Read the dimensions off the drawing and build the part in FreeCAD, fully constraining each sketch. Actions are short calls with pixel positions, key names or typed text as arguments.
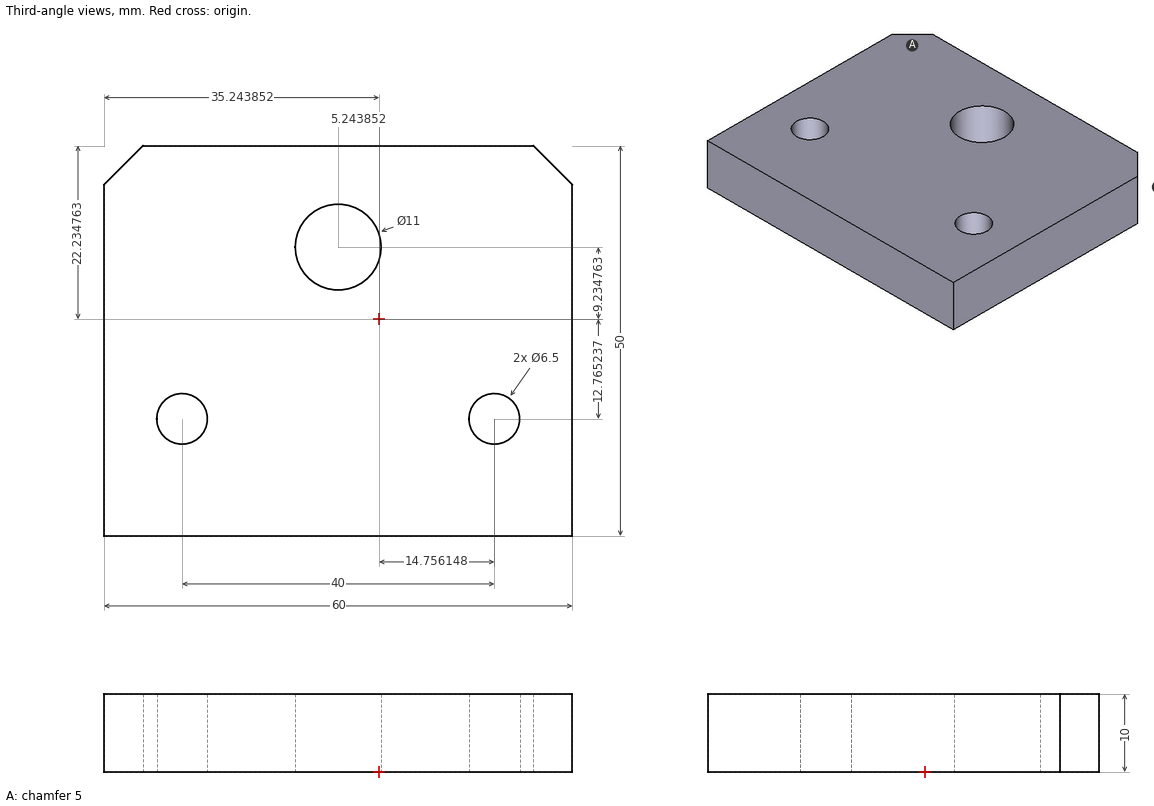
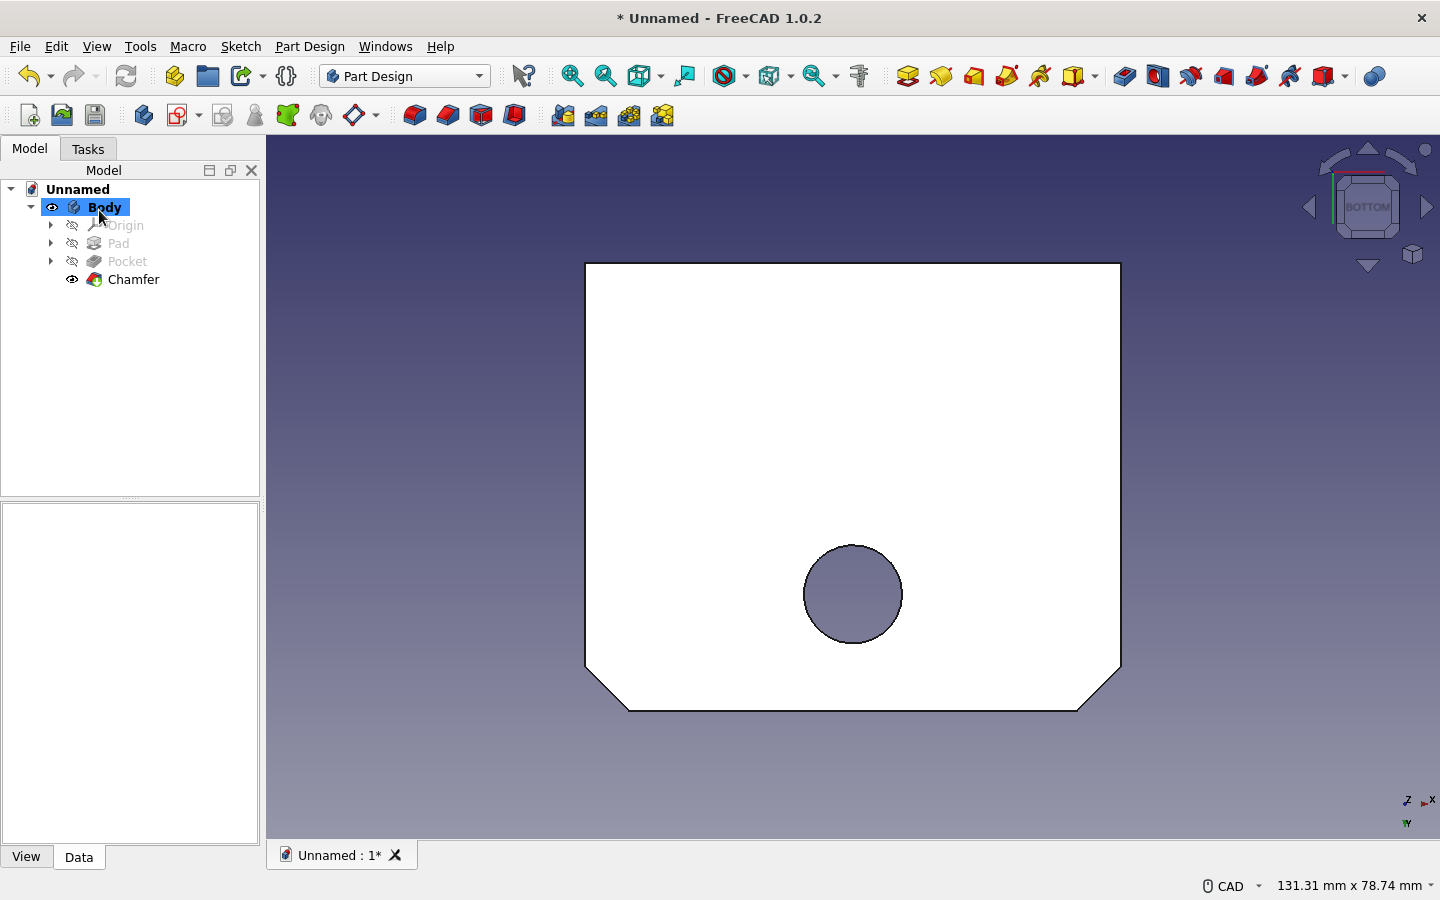
click(776, 422)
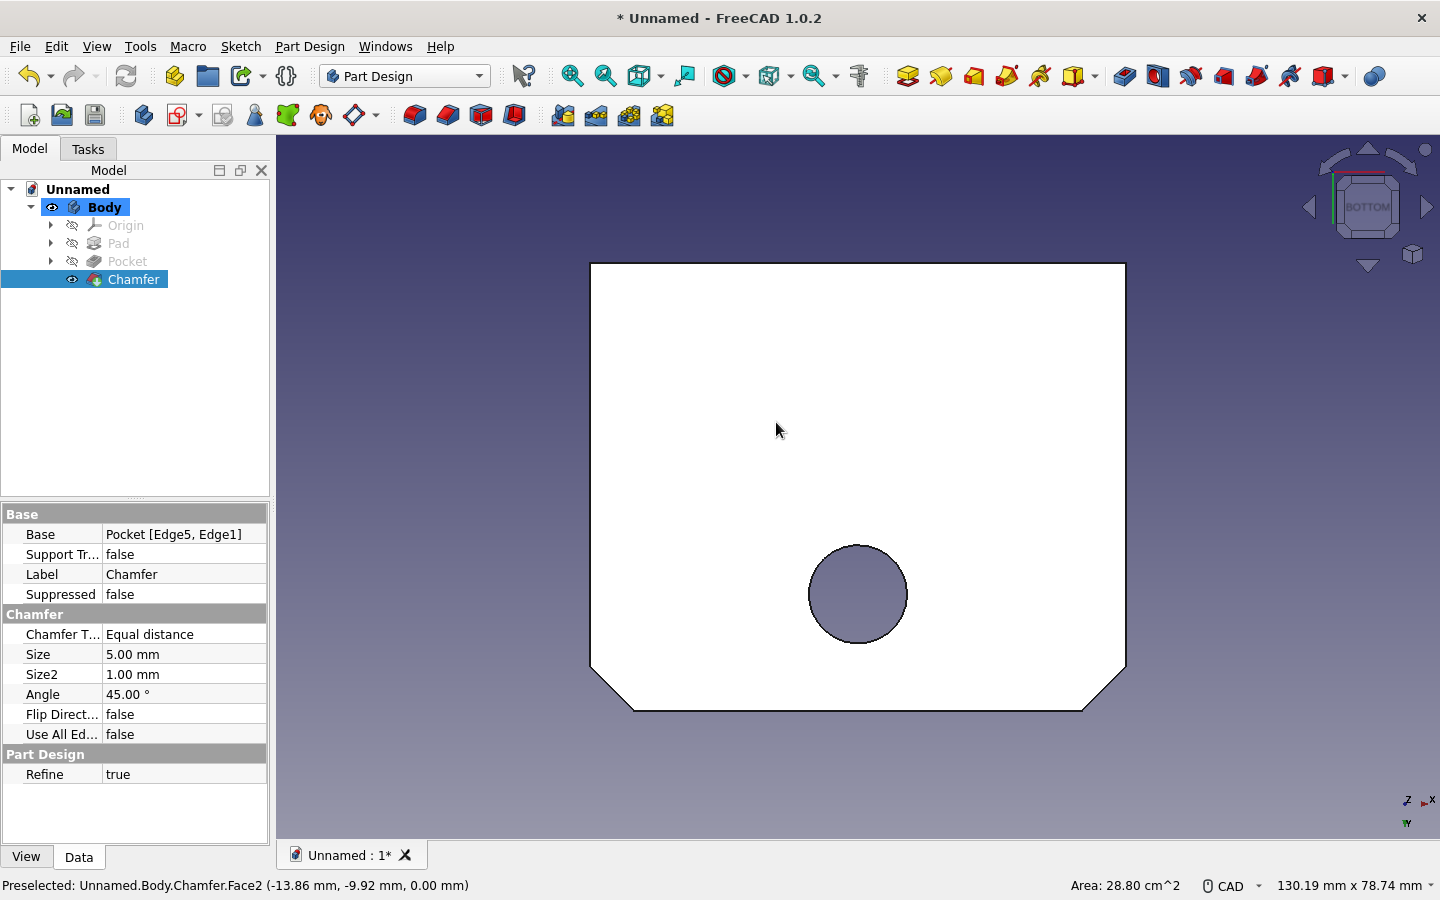
click(176, 116)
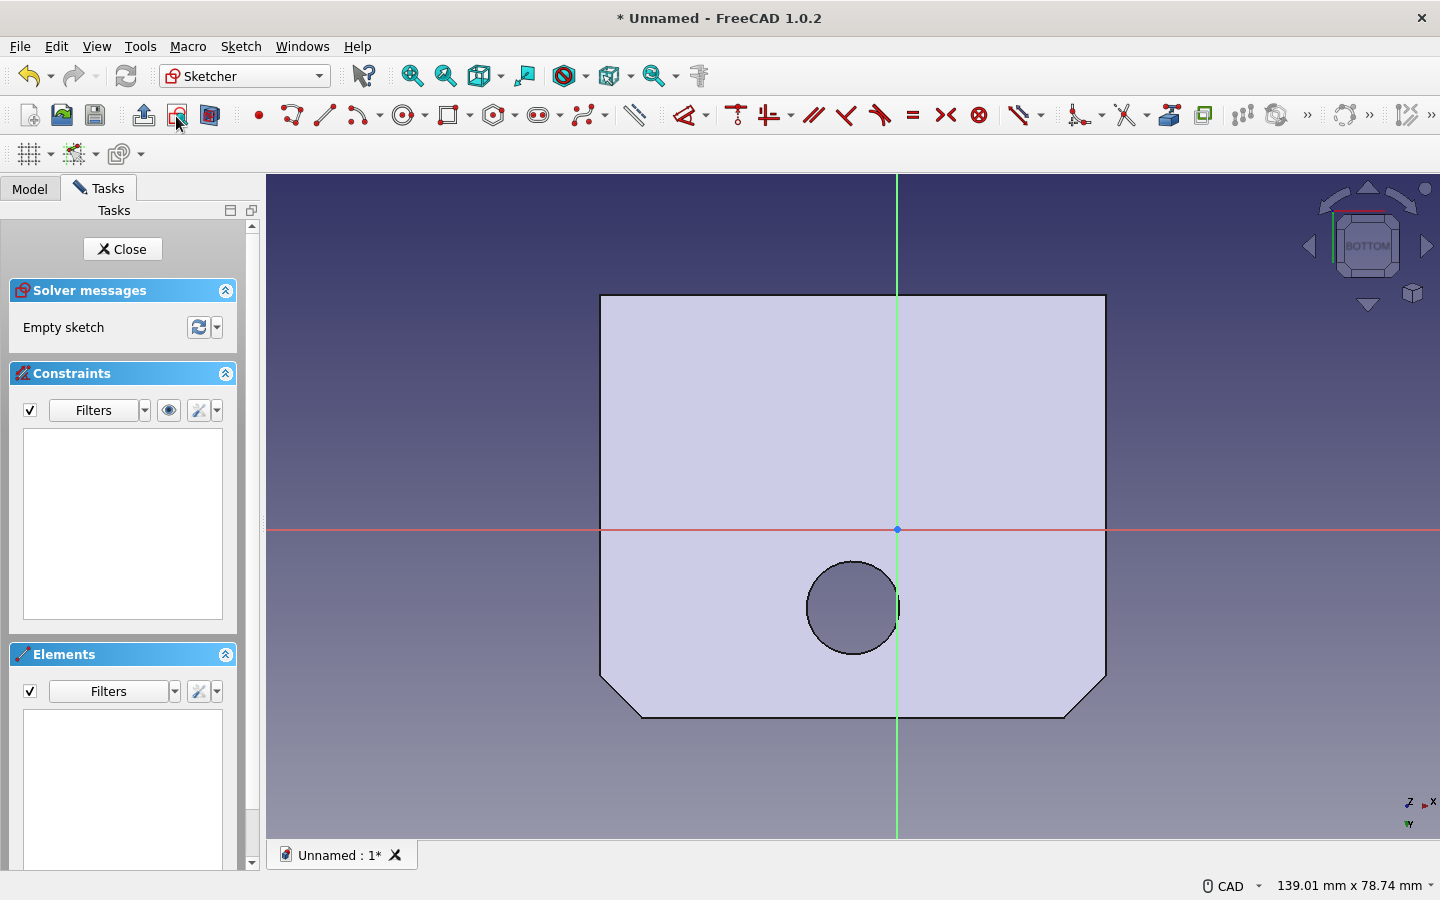
scroll(936, 408, up, 3)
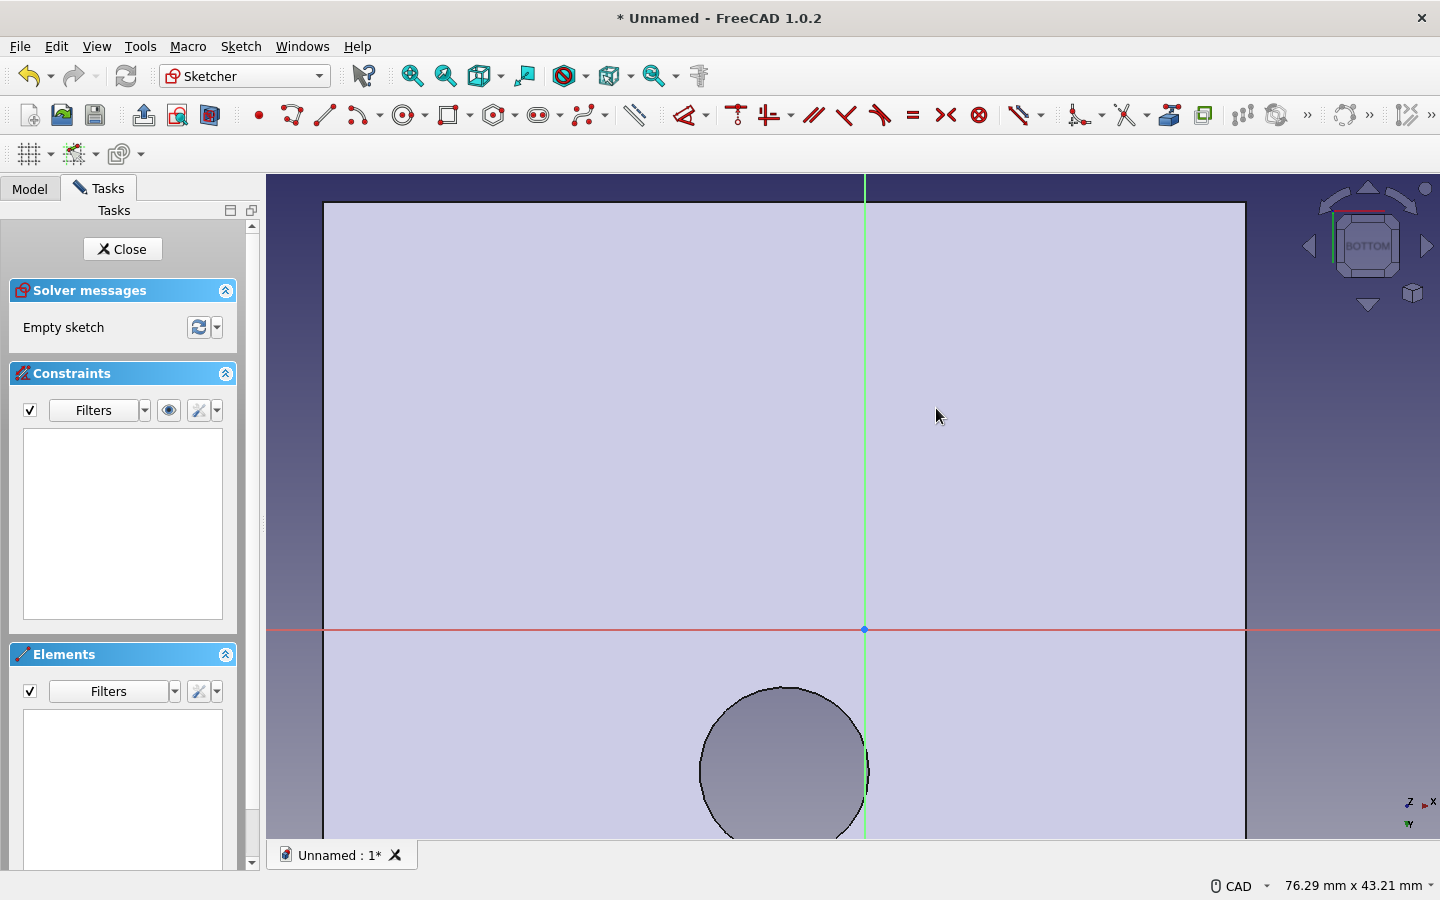
key(g)
key(c)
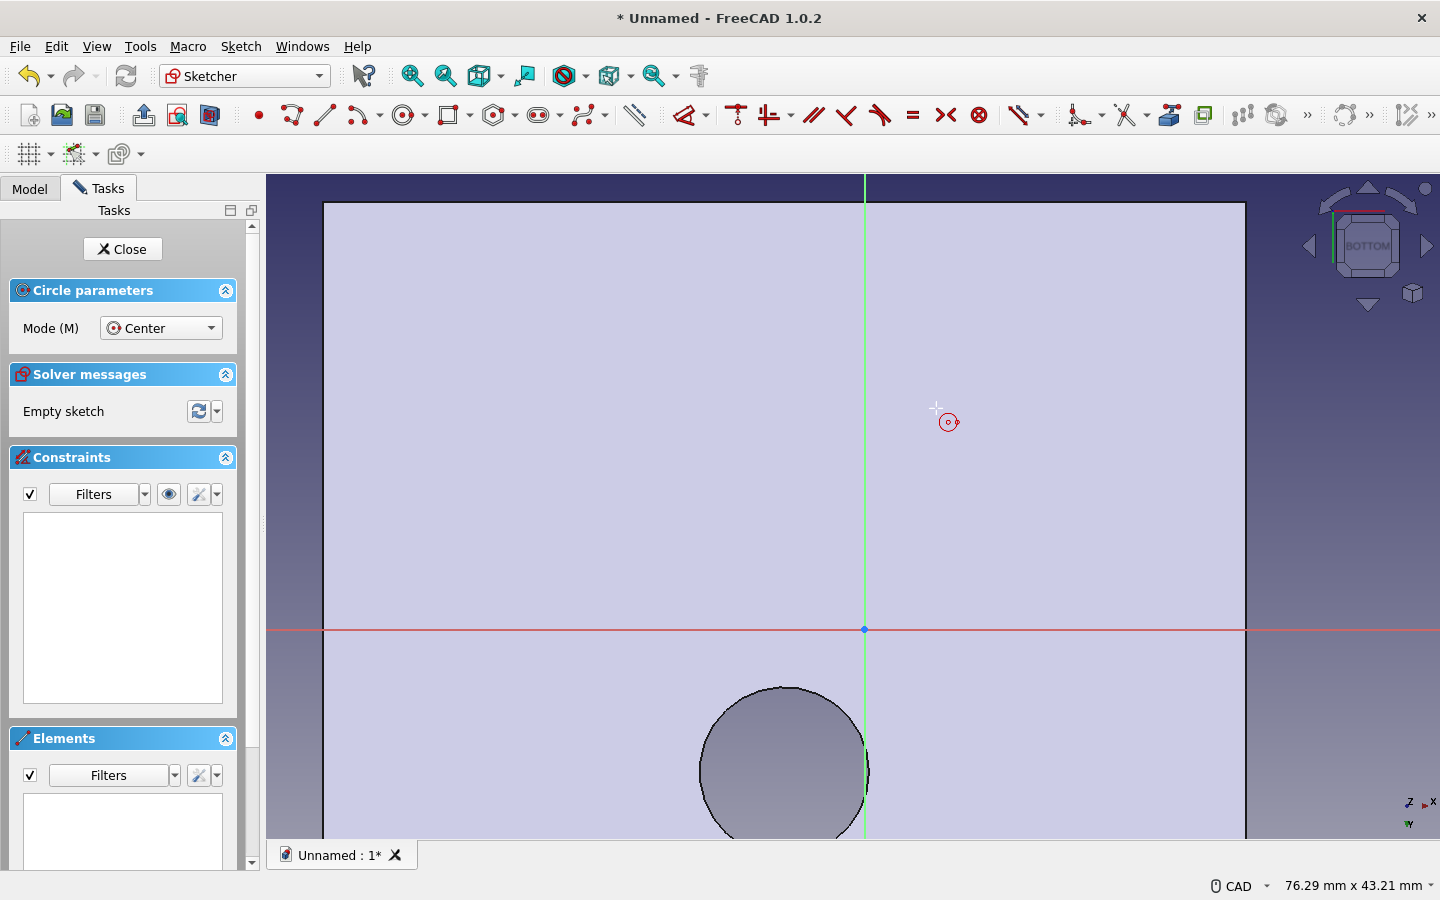
click(1092, 433)
move(1127, 398)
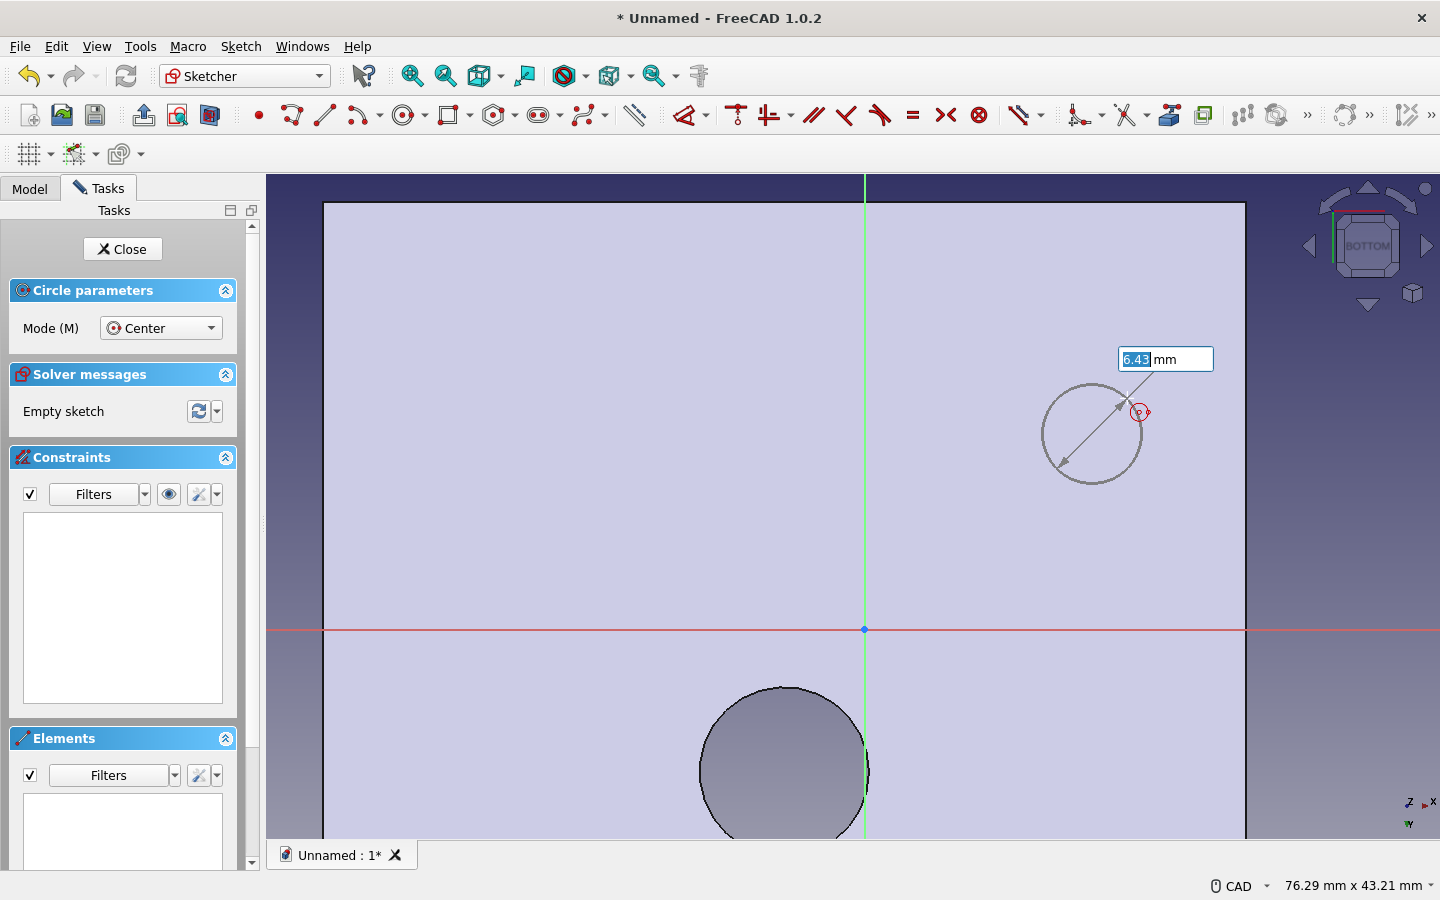
text(6.5)
key(Return)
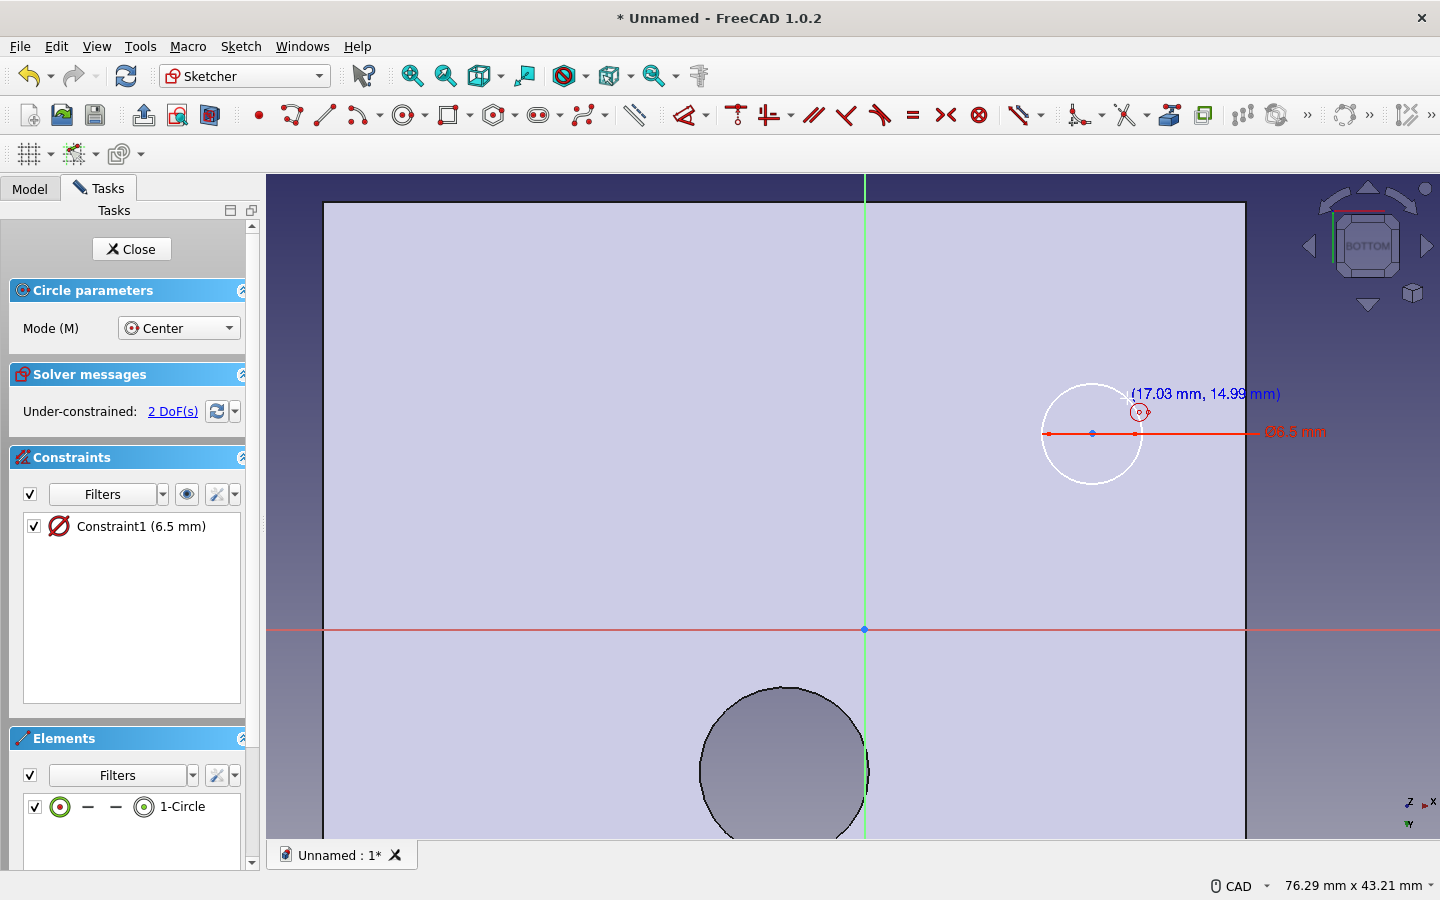
click(477, 433)
move(512, 398)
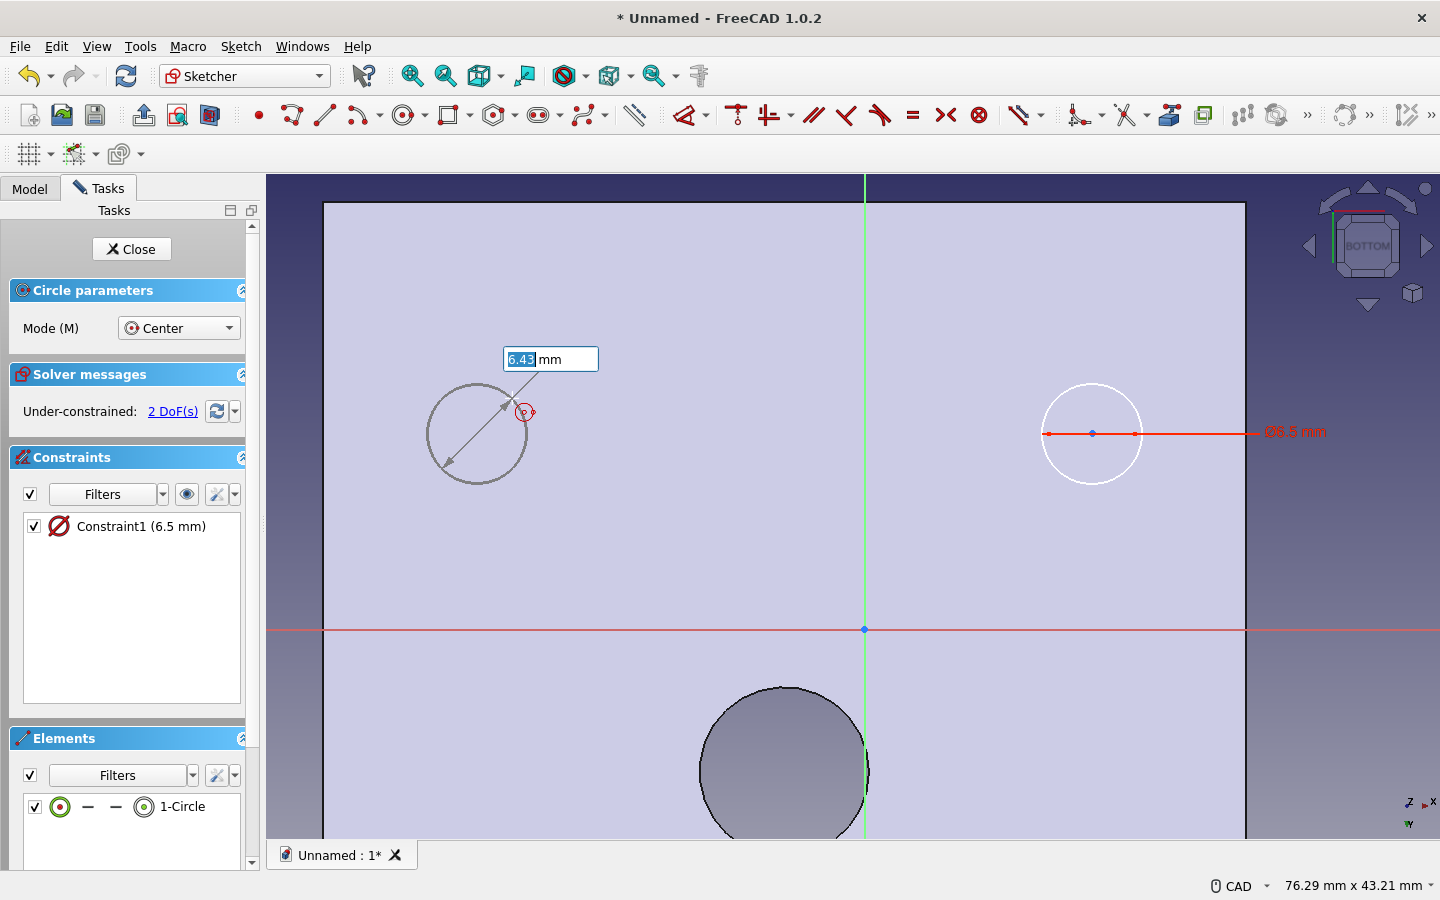
text(6.5)
key(Return)
key(Escape)